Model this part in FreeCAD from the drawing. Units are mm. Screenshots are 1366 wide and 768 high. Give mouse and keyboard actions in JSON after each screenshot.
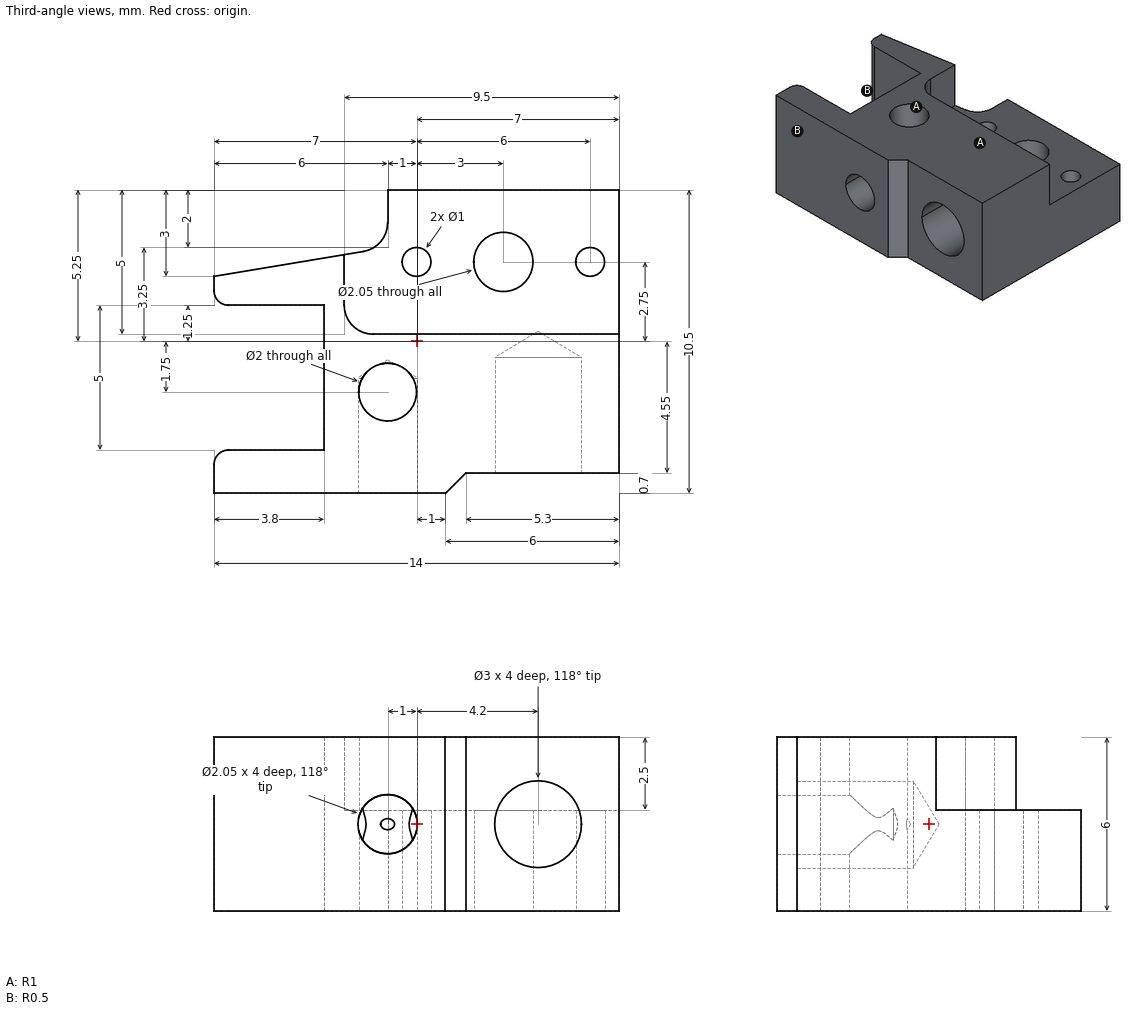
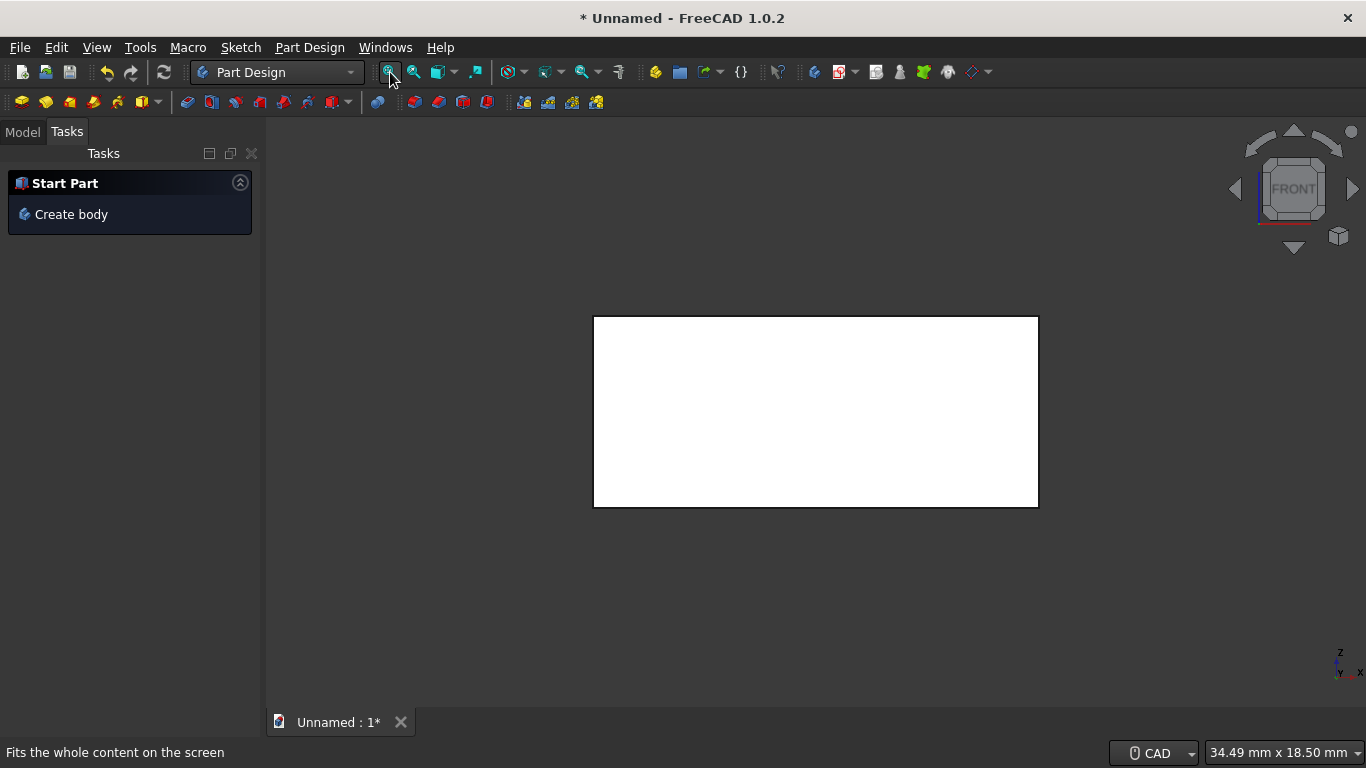
{"action": "key", "text": "3"}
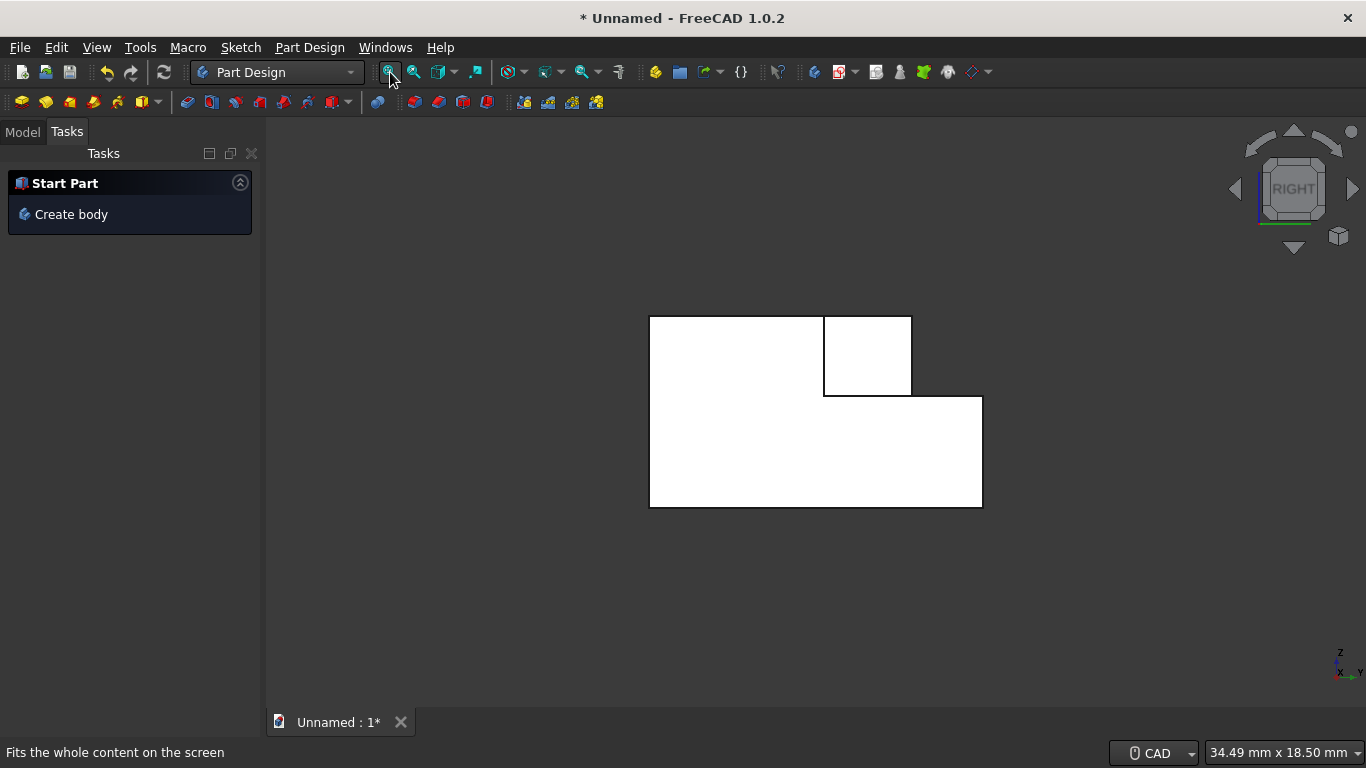
{"action": "left_click", "coordinate": [390, 72]}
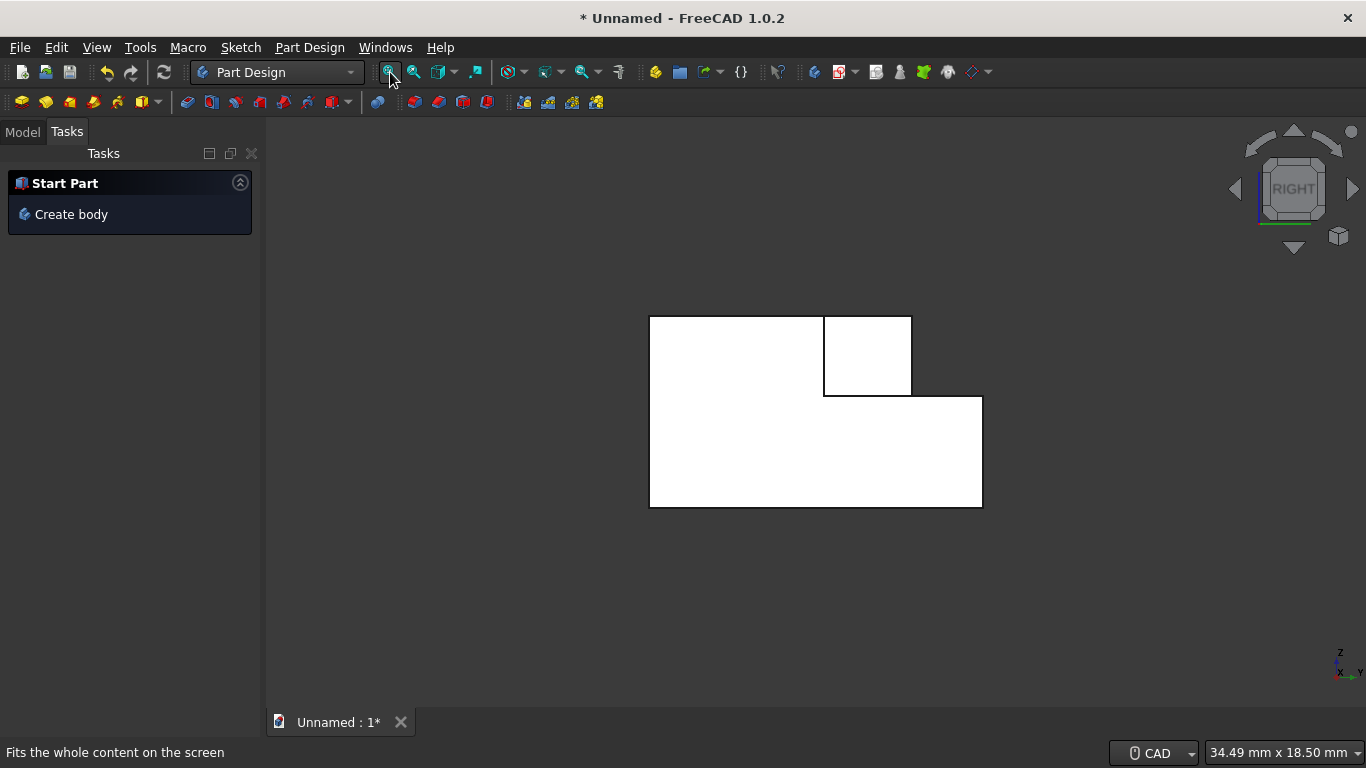
{"action": "key", "text": "5"}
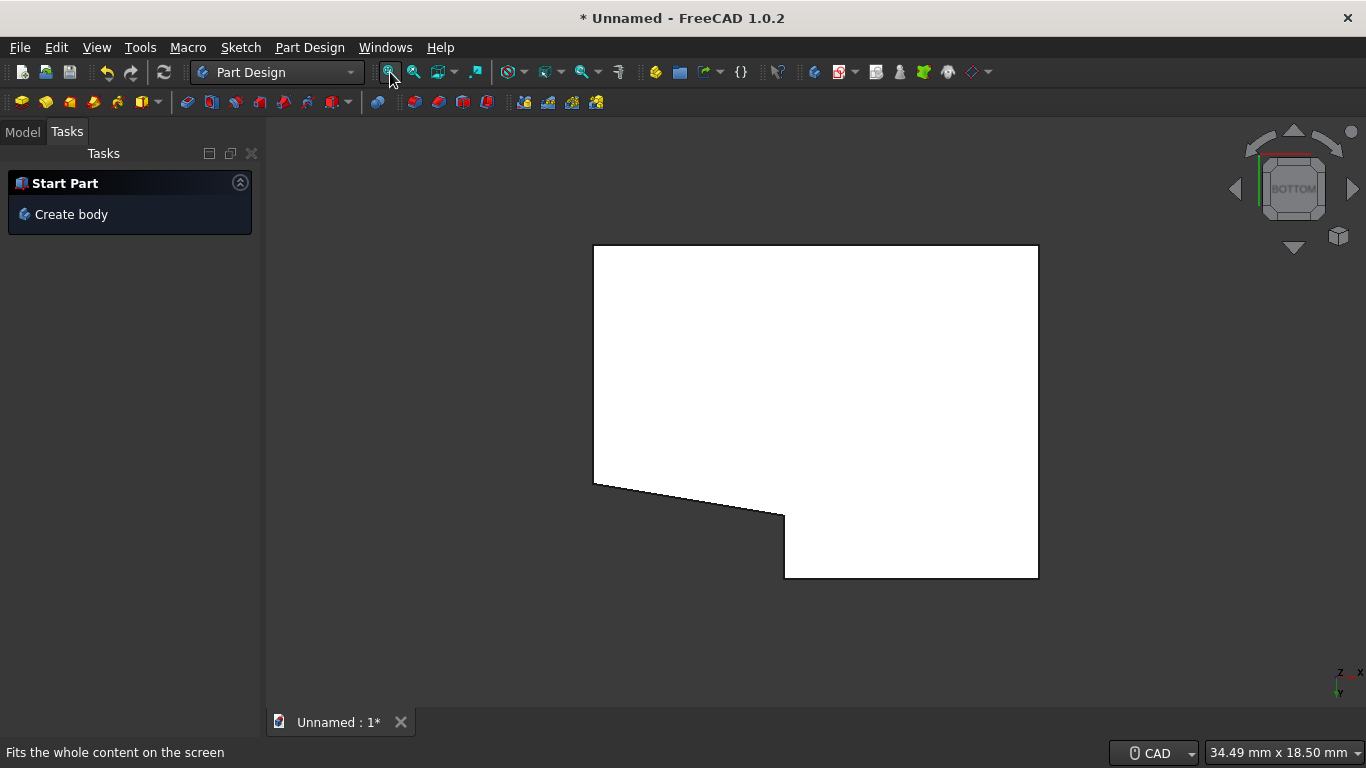
{"action": "key", "text": "4"}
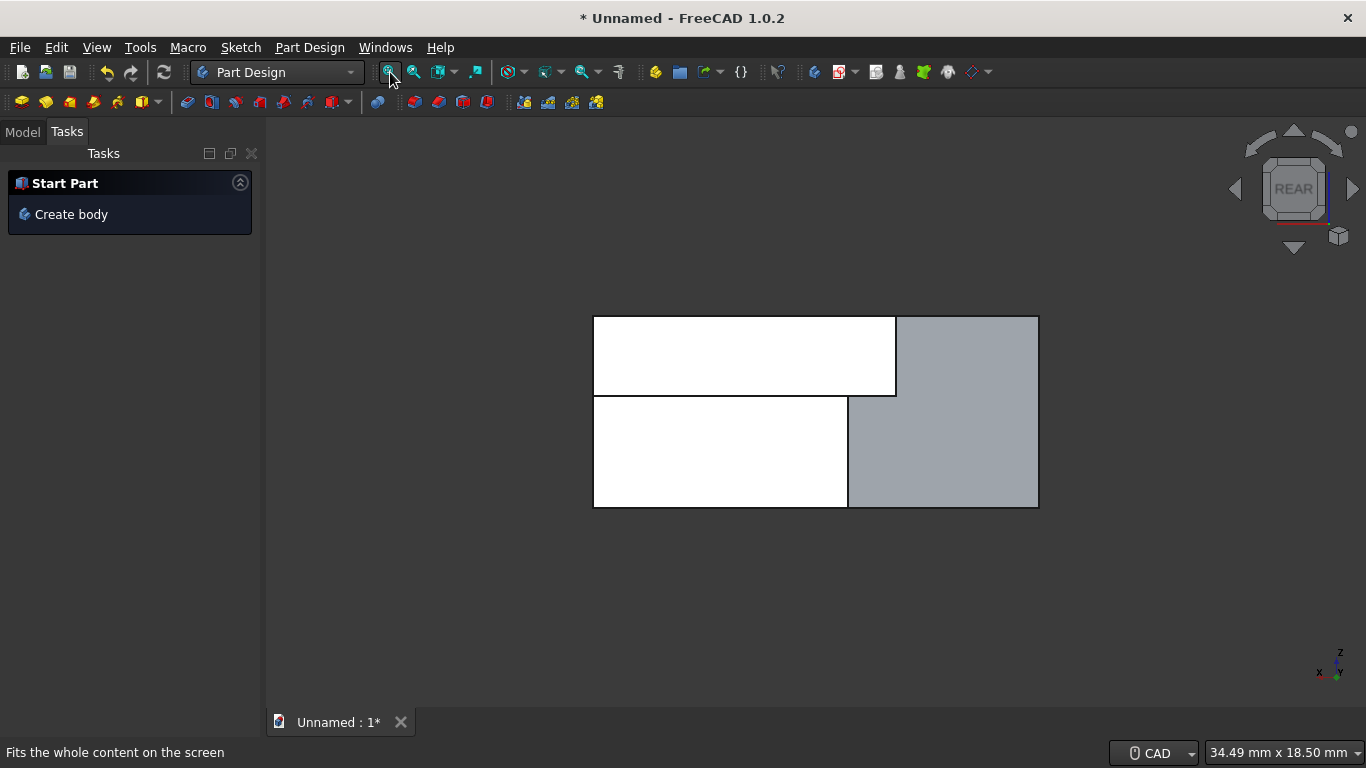
{"action": "left_click", "coordinate": [390, 72]}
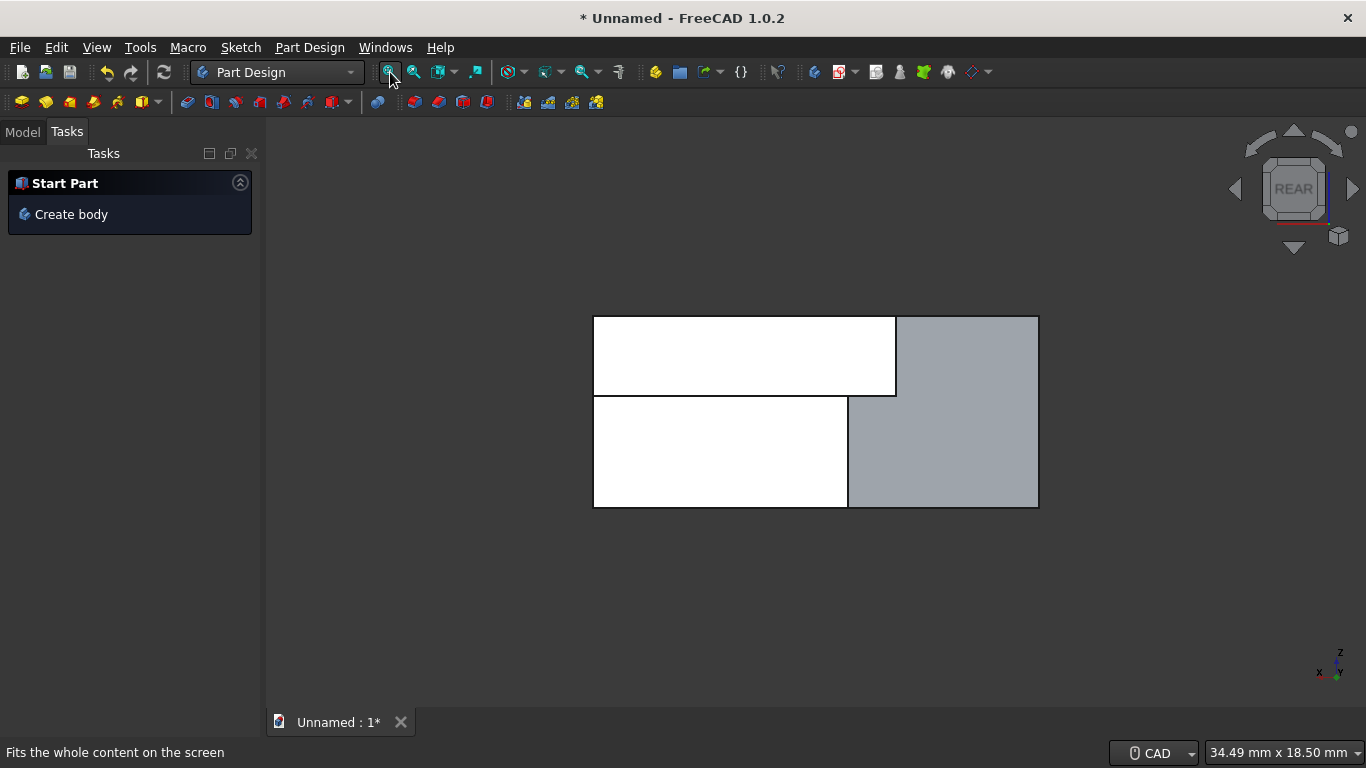
{"action": "key", "text": "6"}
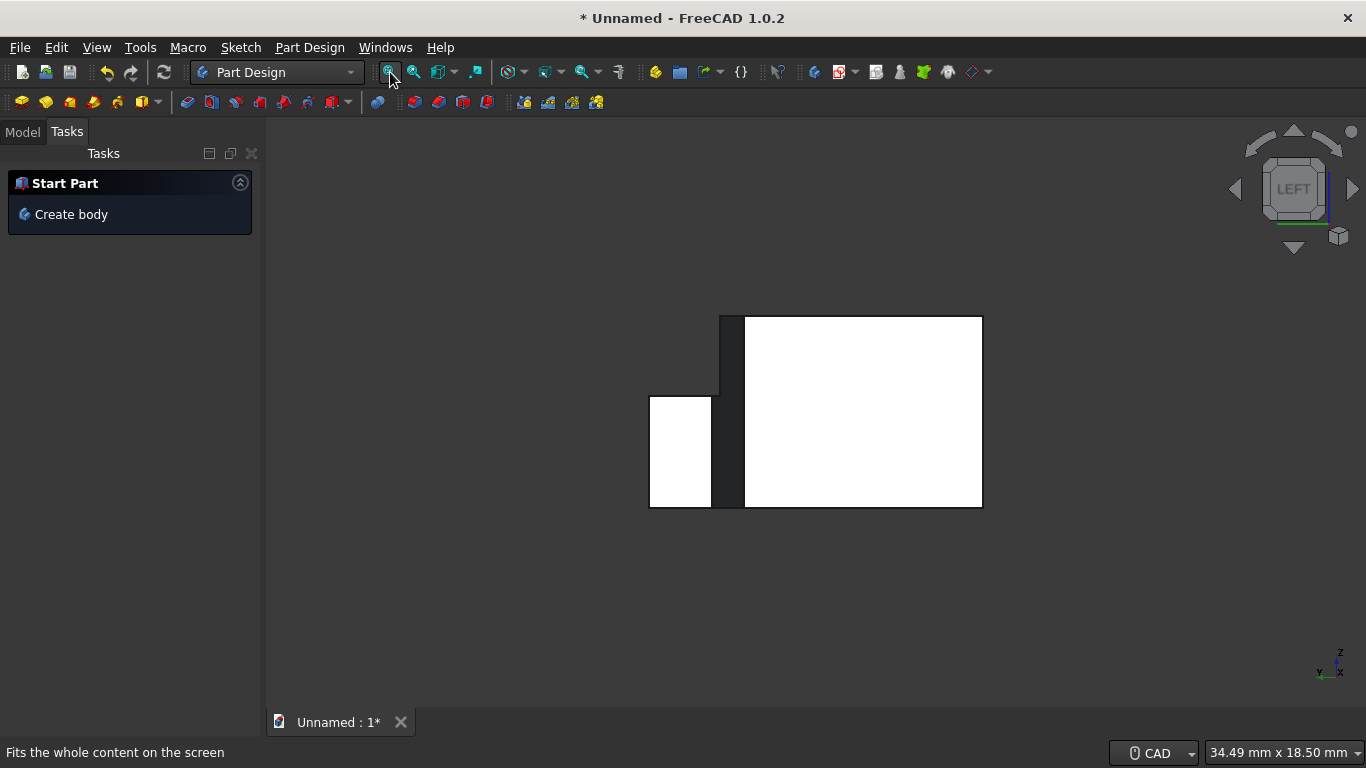
{"action": "left_click", "coordinate": [390, 72]}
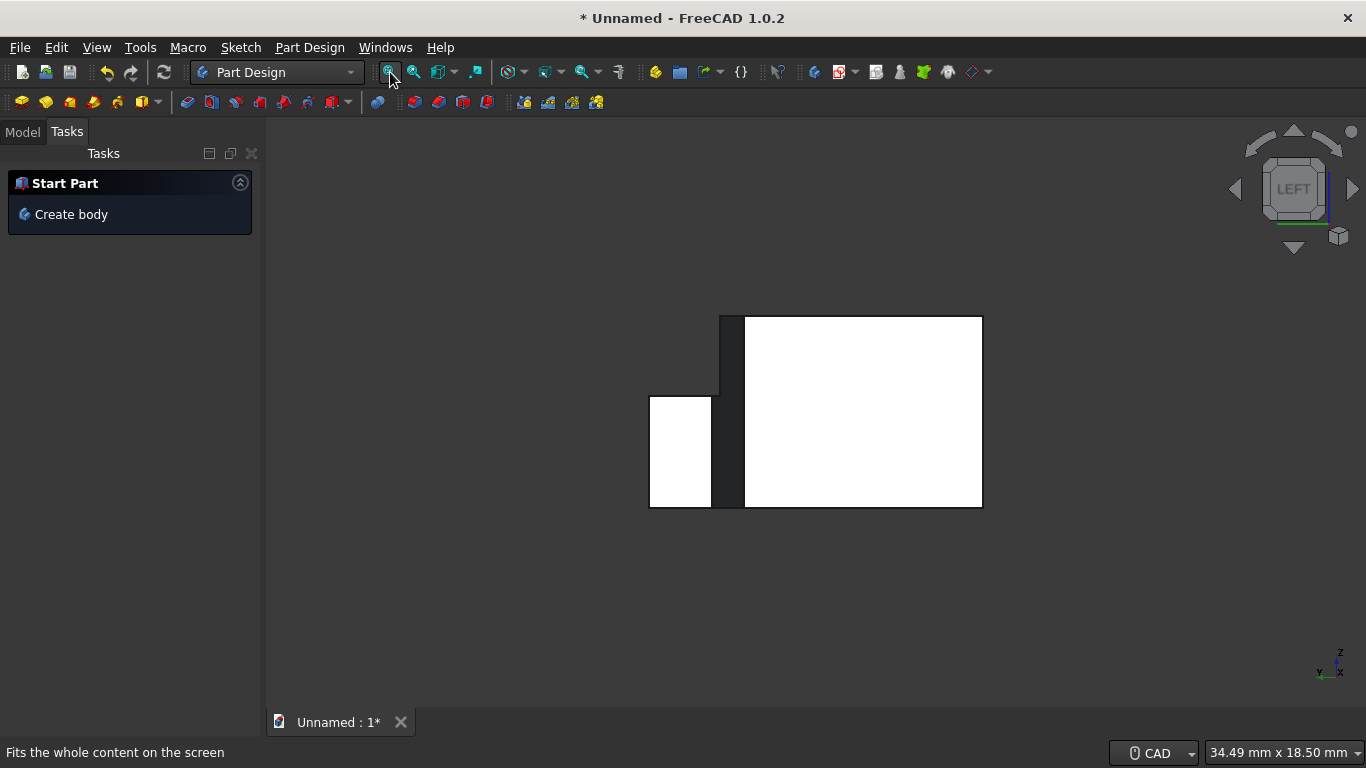
{"action": "key", "text": "v 3"}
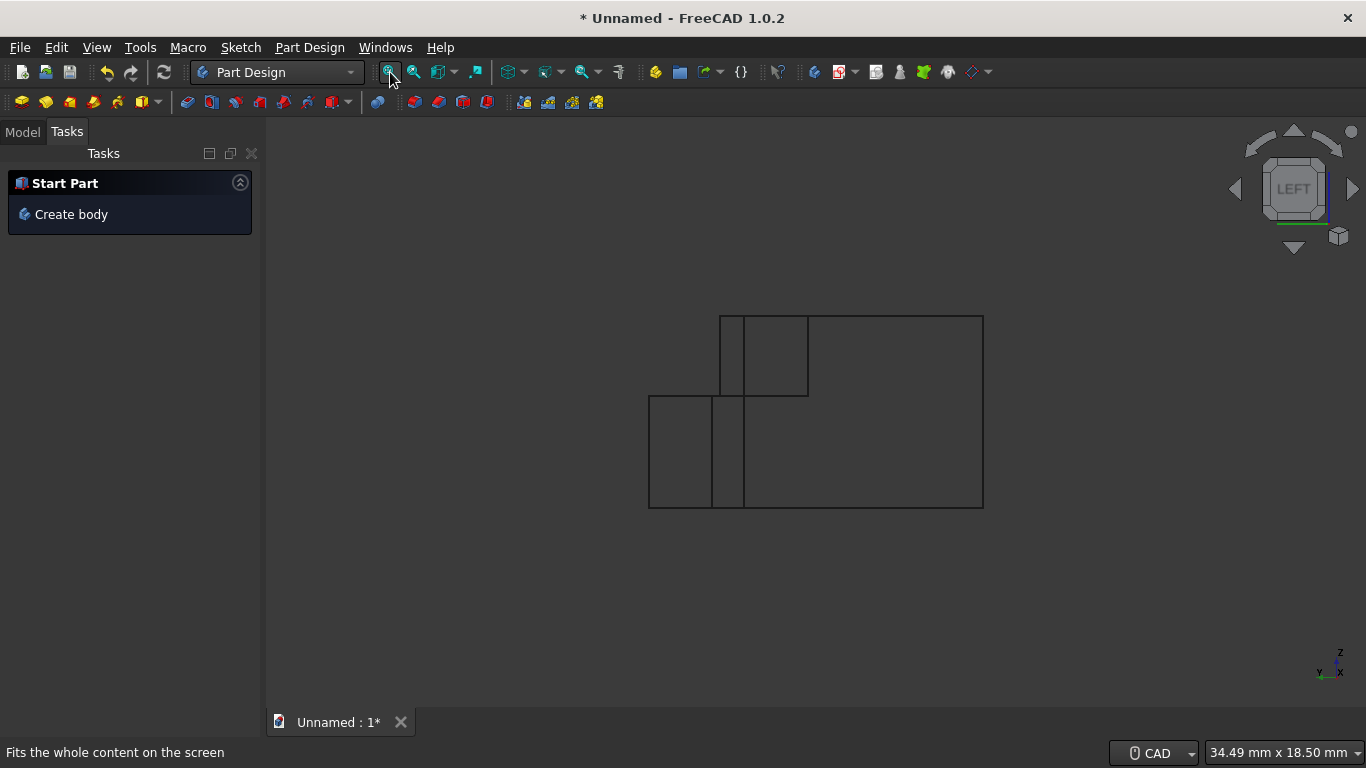
{"action": "key", "text": "0"}